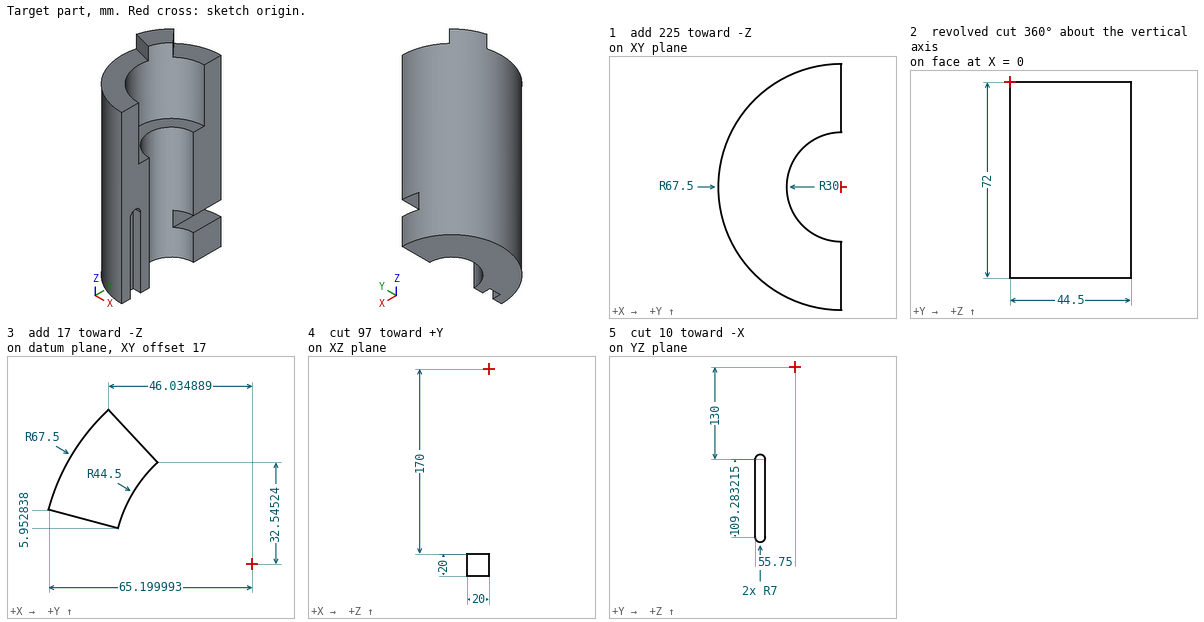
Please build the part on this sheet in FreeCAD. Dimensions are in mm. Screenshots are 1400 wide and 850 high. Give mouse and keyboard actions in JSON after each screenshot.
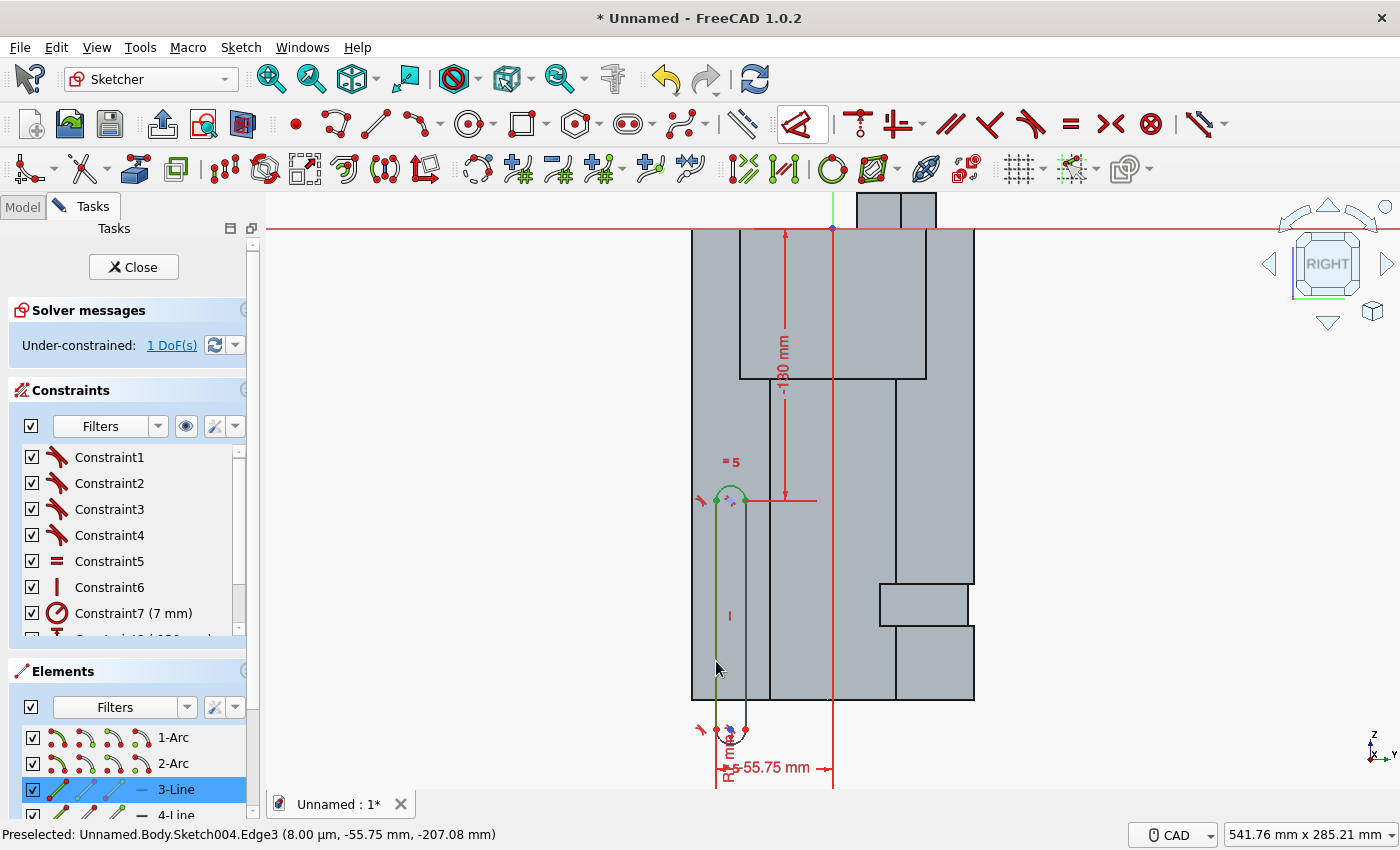
{"action": "key", "text": "i"}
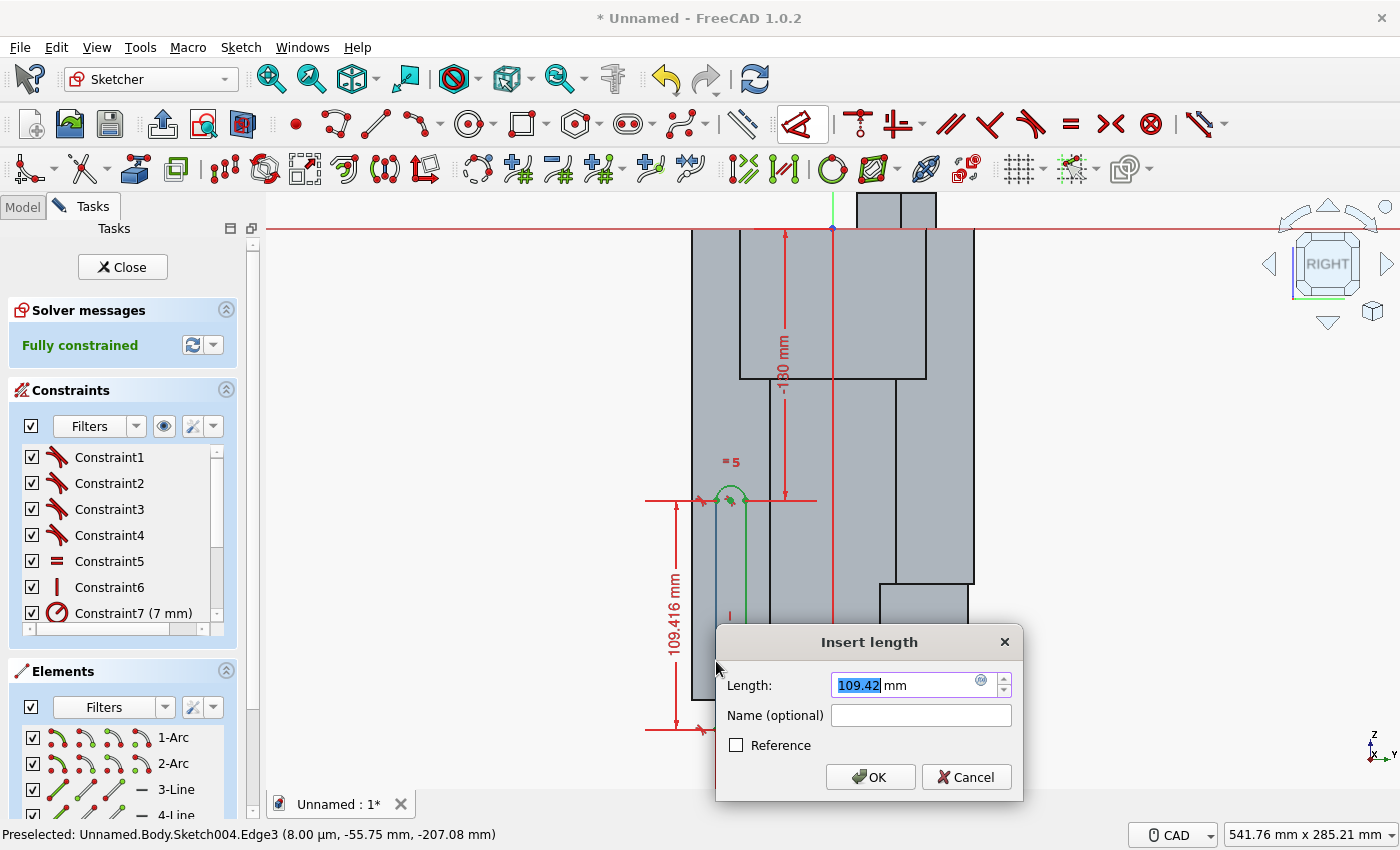
{"action": "type", "text": "109.283215"}
{"action": "key", "text": "Return"}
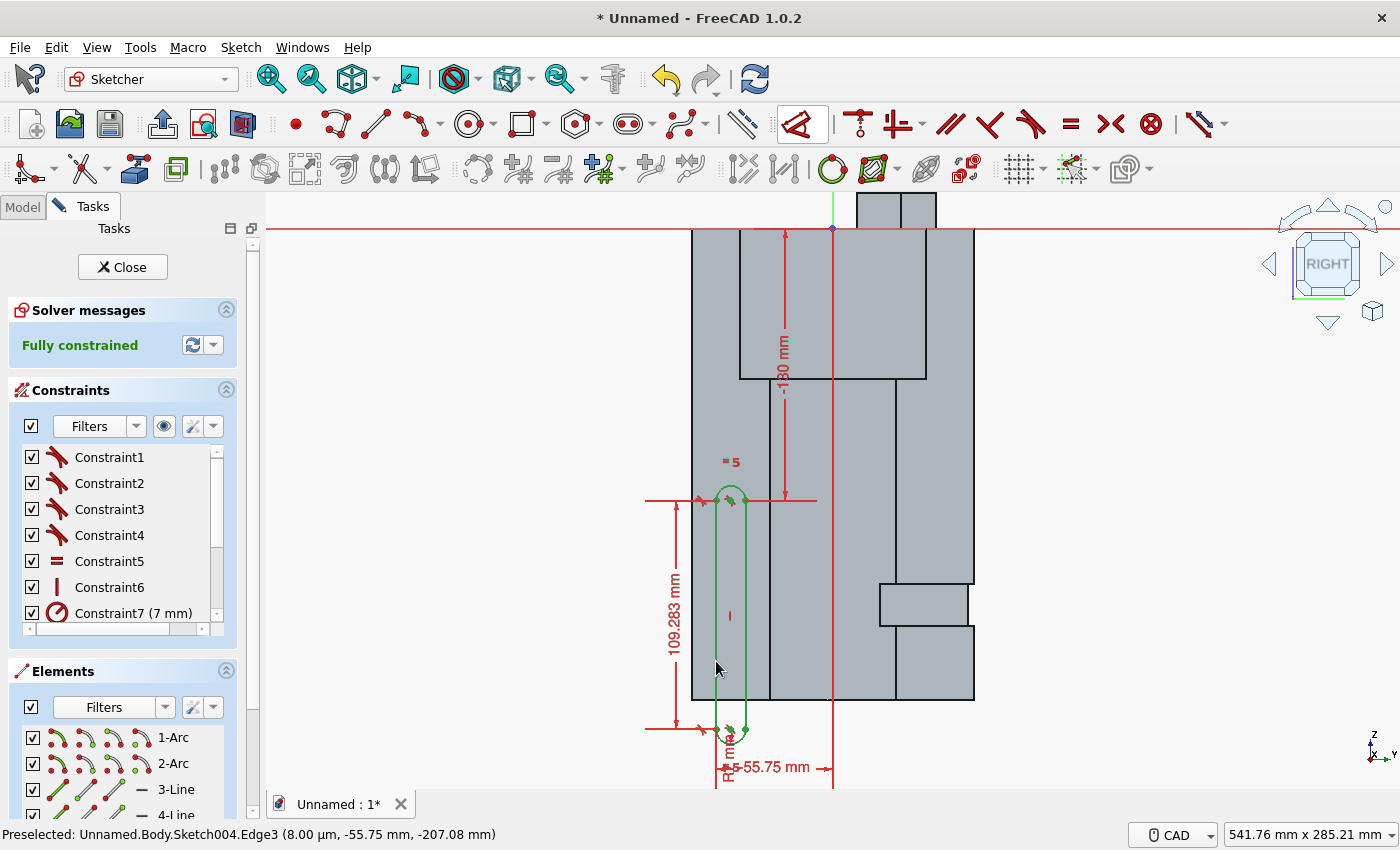
{"action": "left_click", "coordinate": [123, 267]}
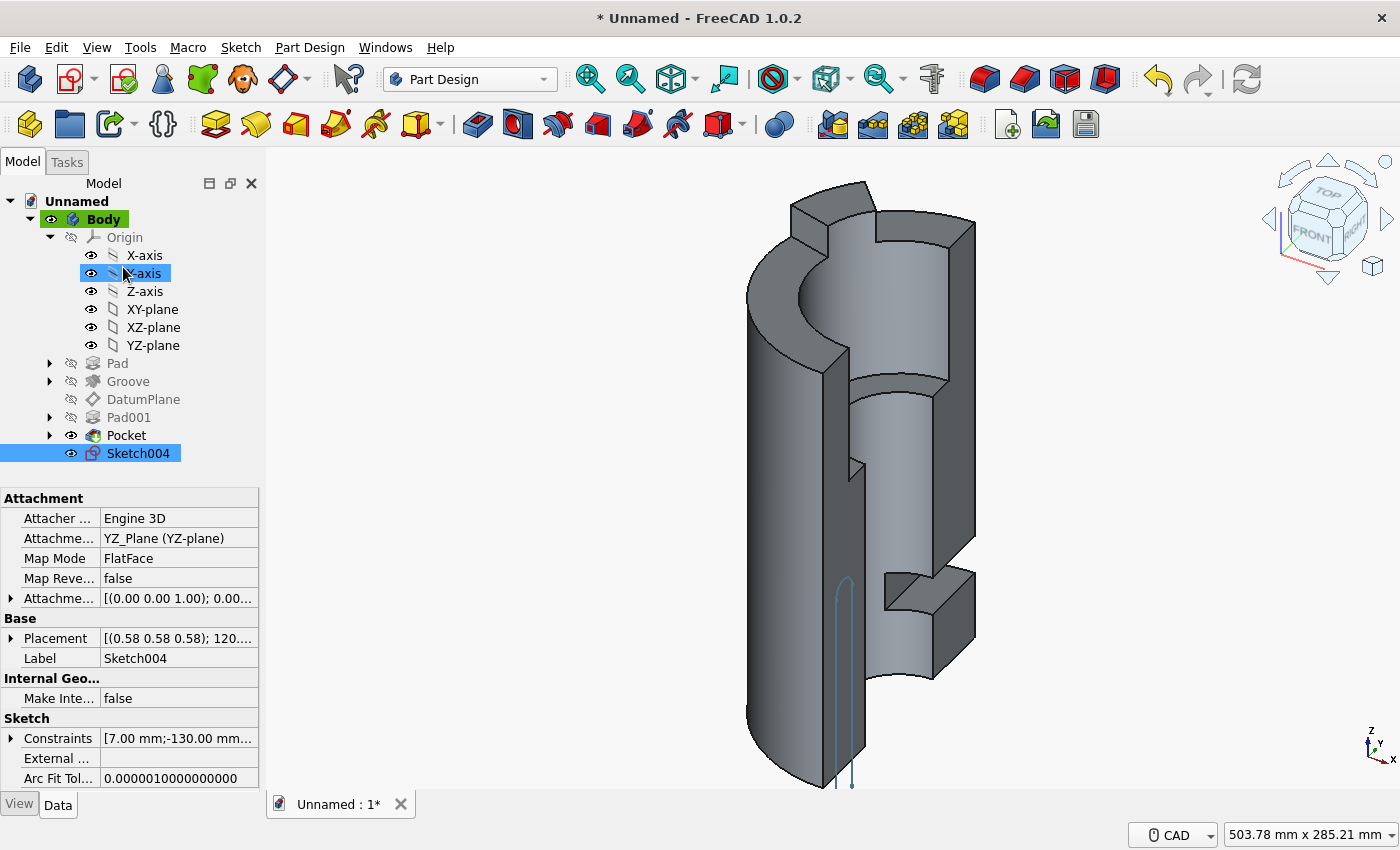
{"action": "left_click", "coordinate": [478, 124]}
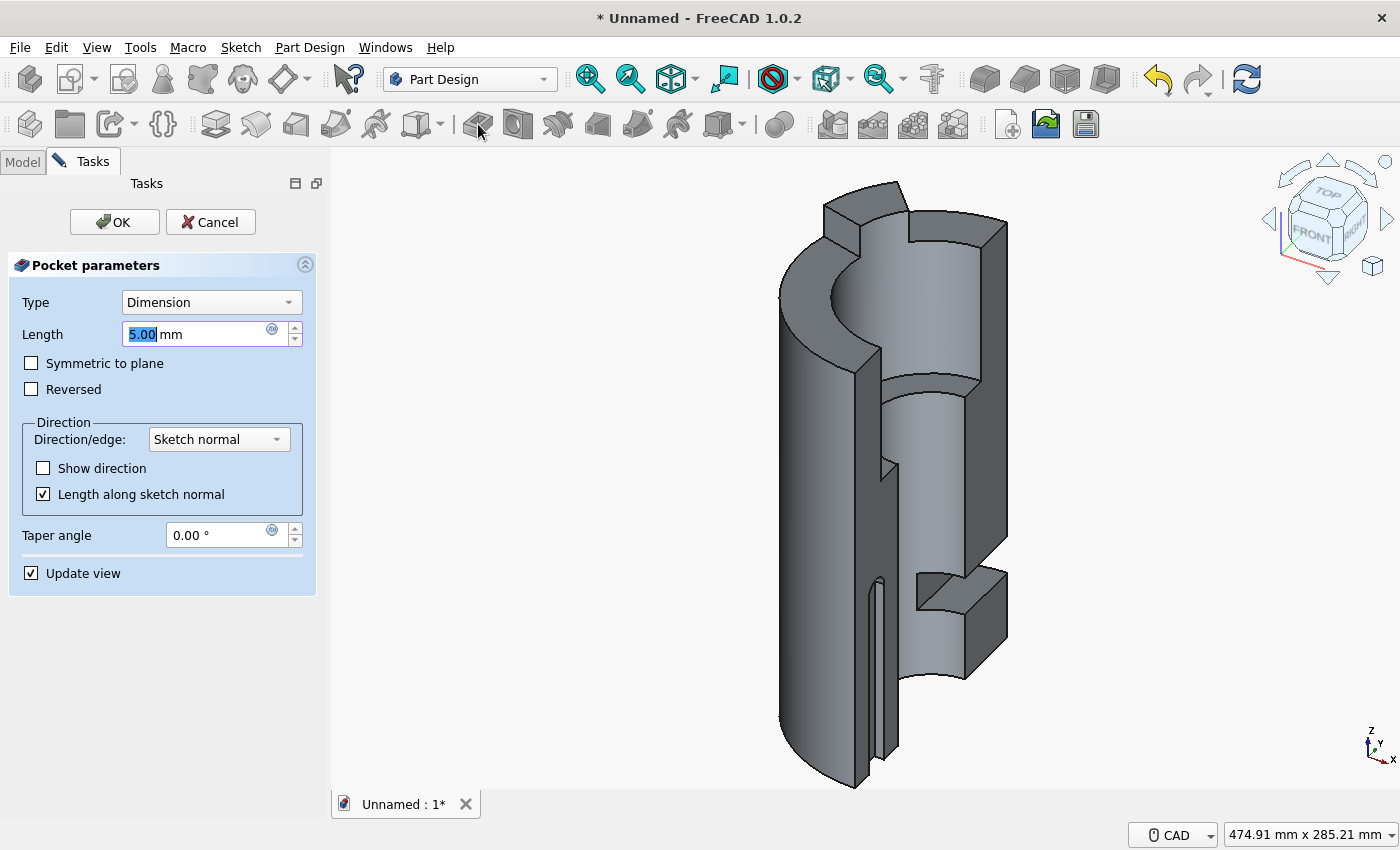
{"action": "type", "text": "10"}
{"action": "key", "text": "Tab"}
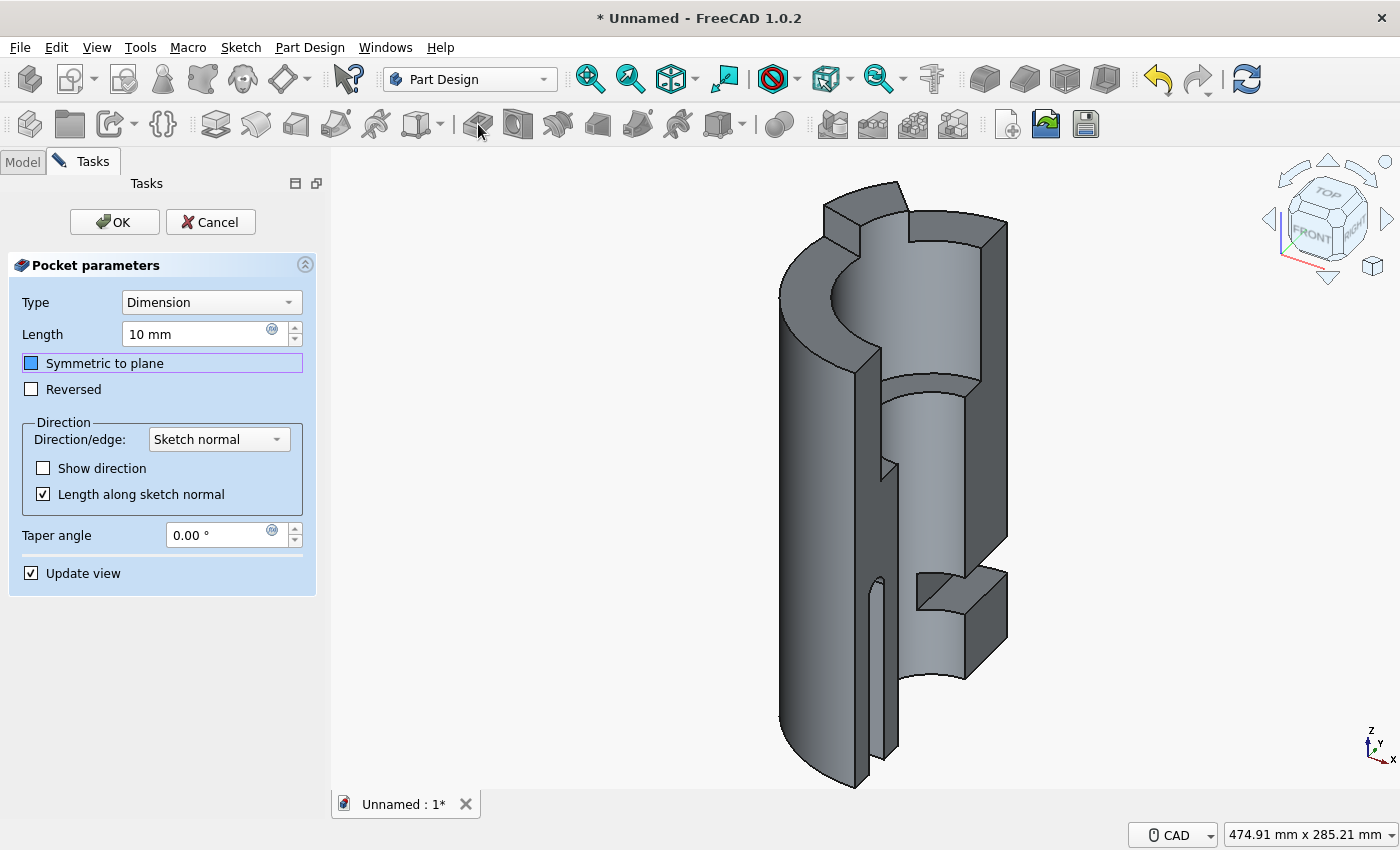
{"action": "left_click", "coordinate": [115, 222]}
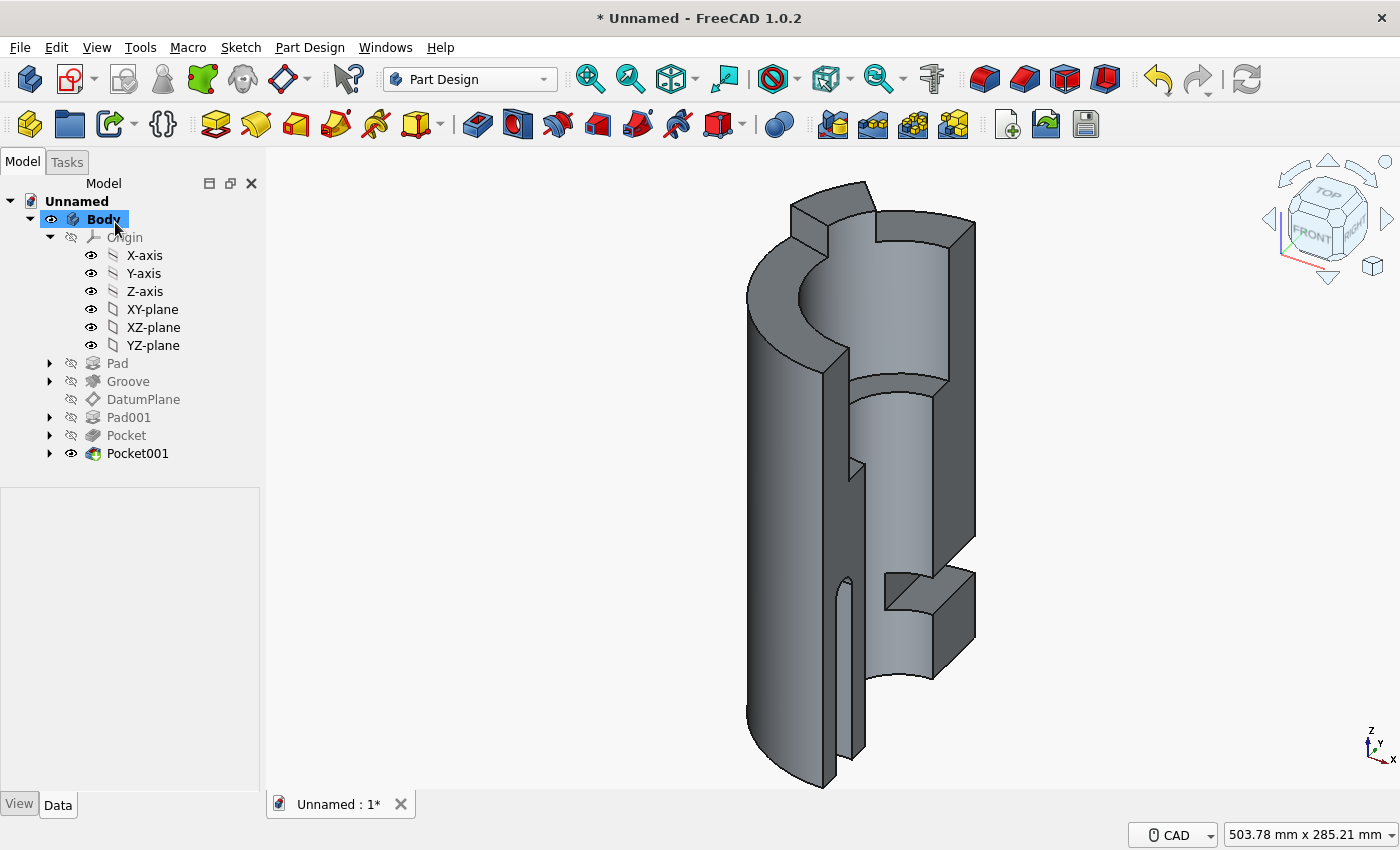
{"action": "key", "text": "0"}